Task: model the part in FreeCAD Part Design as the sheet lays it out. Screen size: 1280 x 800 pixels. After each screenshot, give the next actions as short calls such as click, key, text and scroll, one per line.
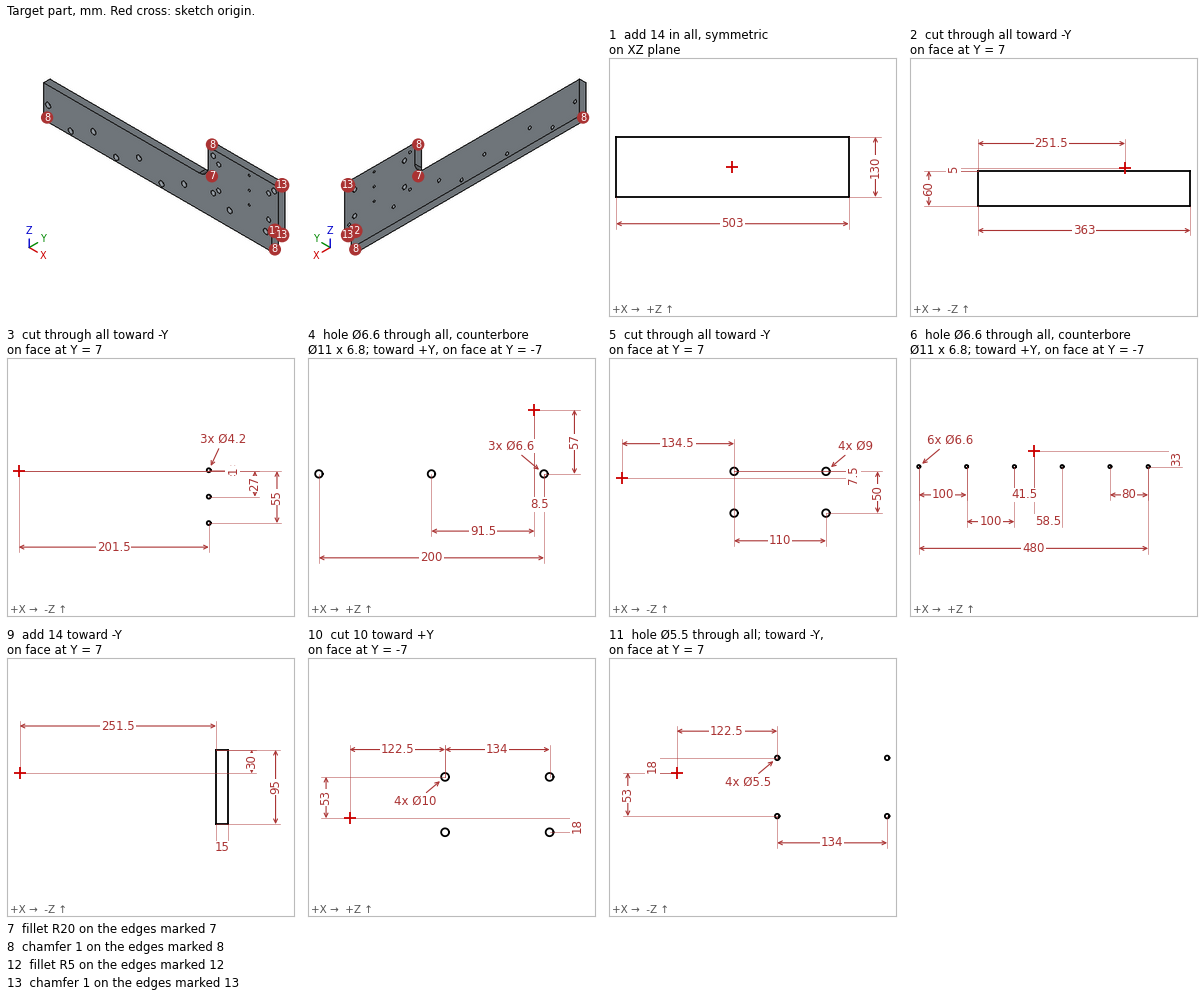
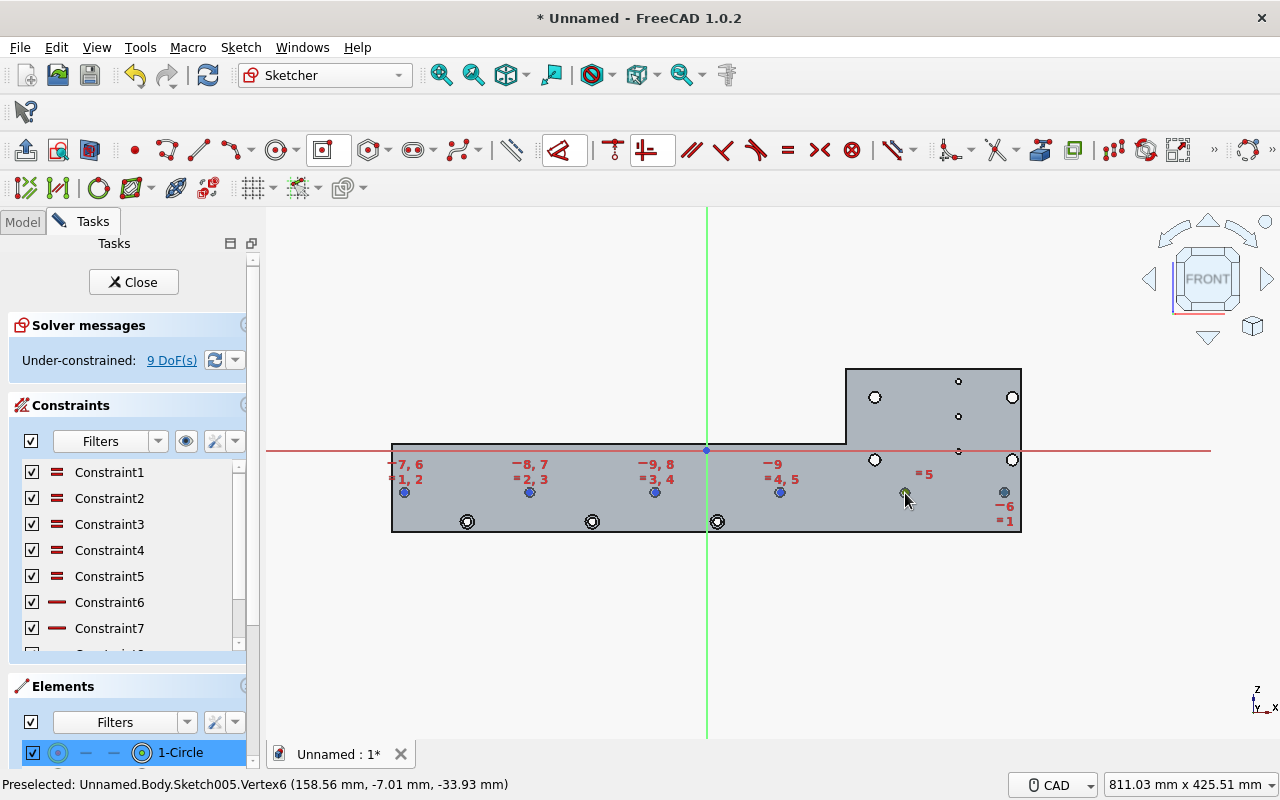
key(h)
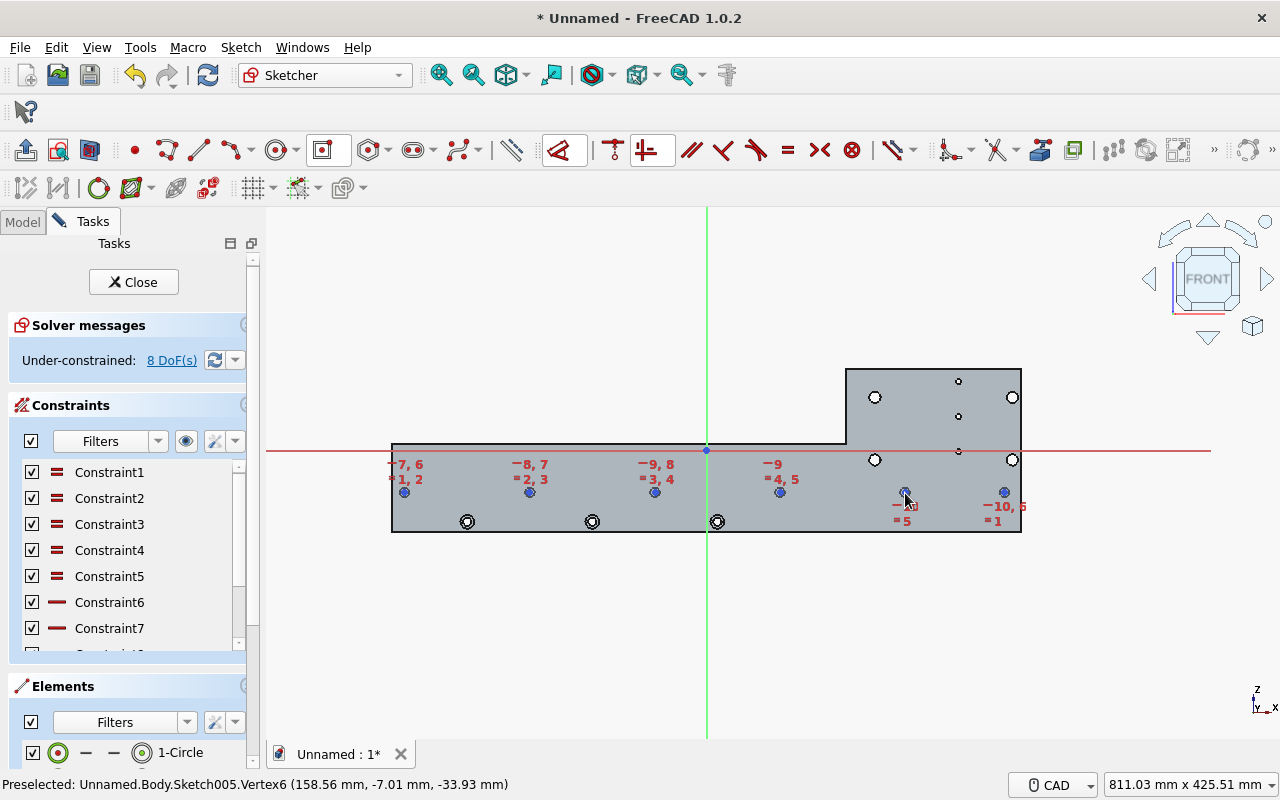
scroll(1000, 492, up, 8)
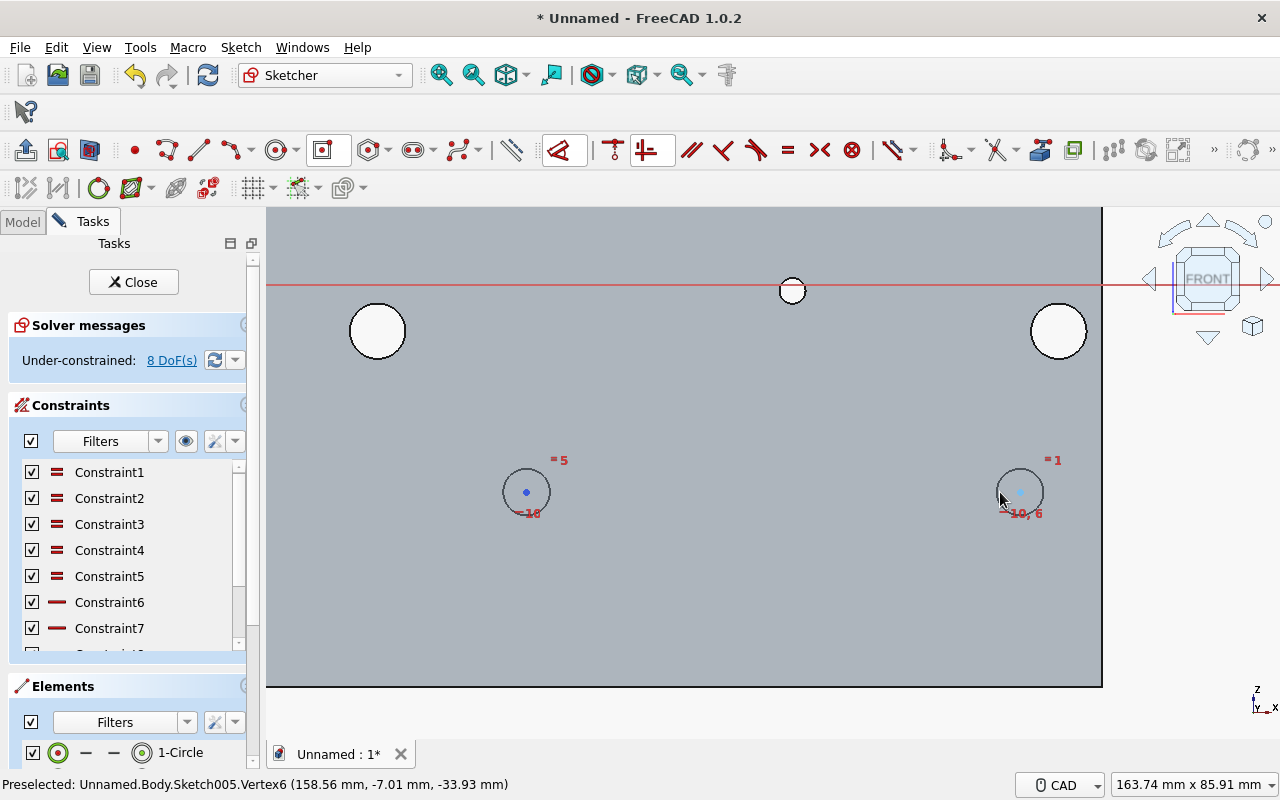
click(997, 491)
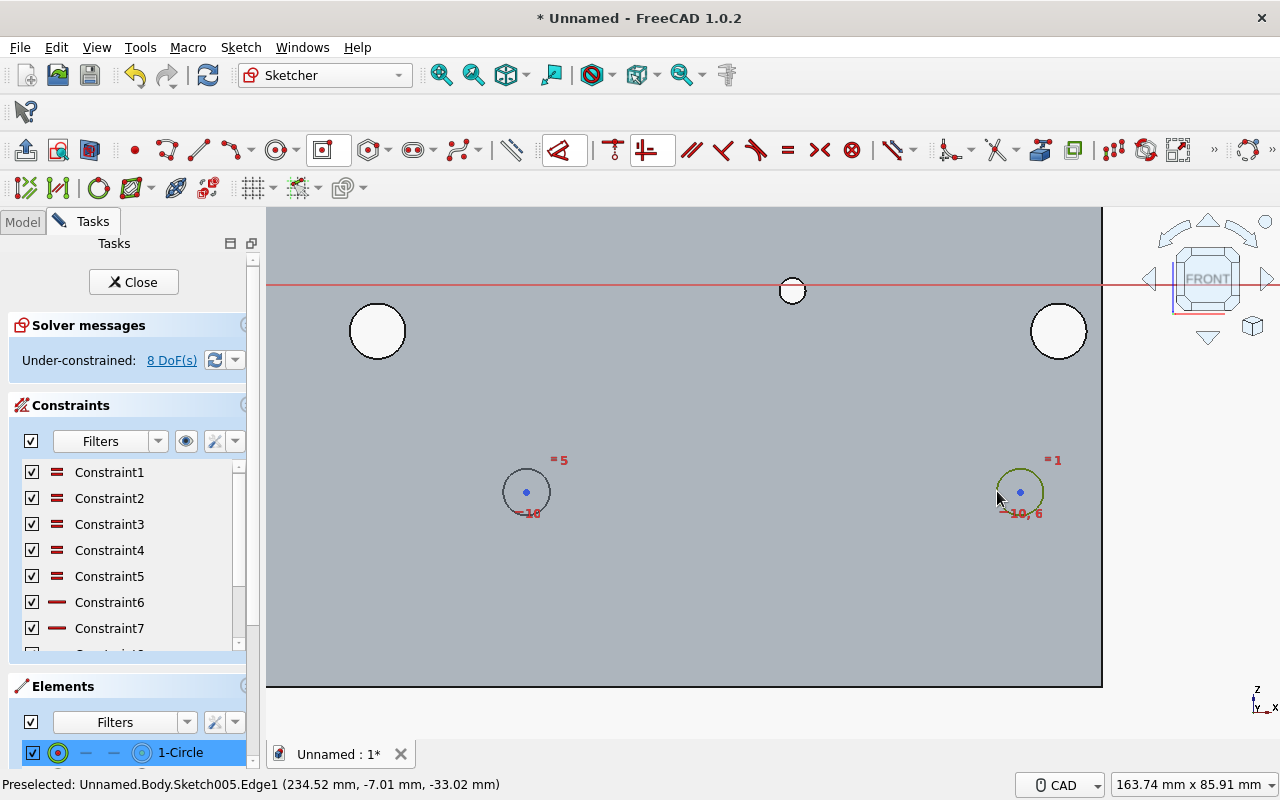
key(k)
key(o)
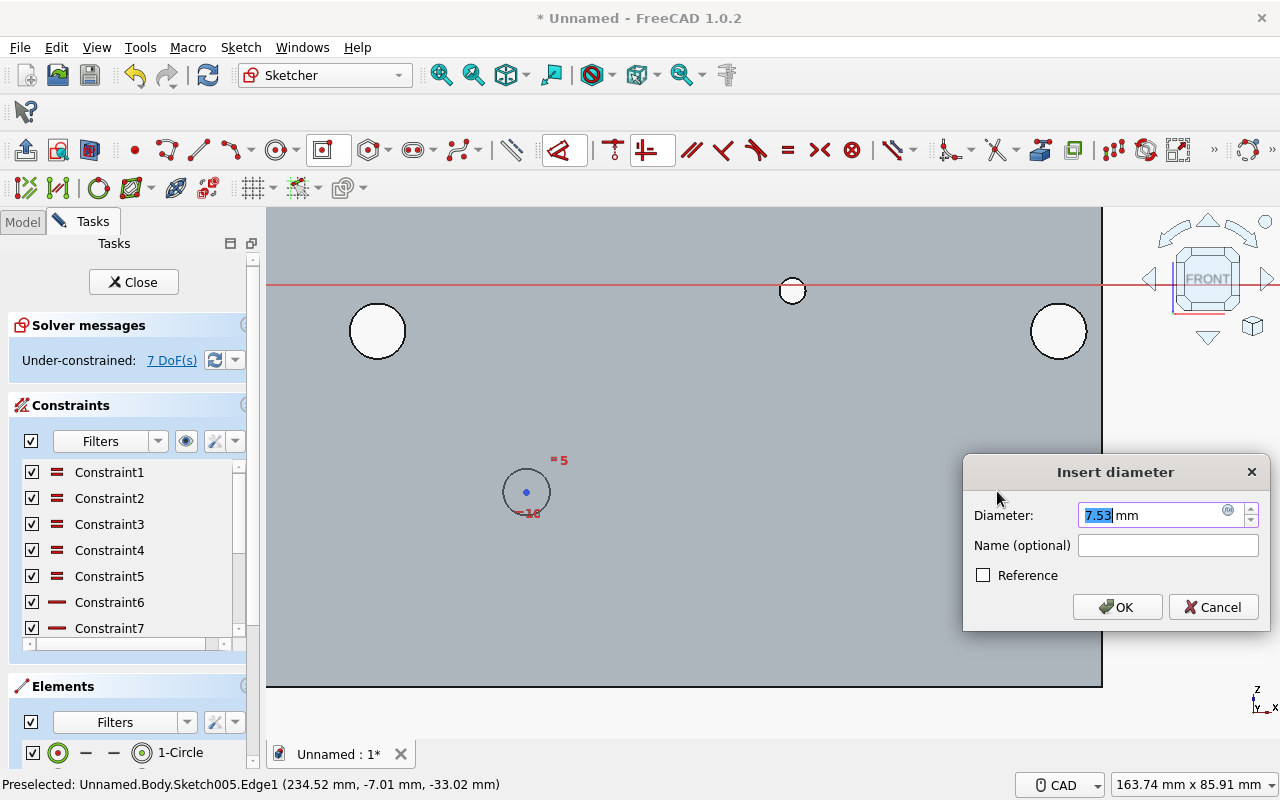
text(6.6)
key(Return)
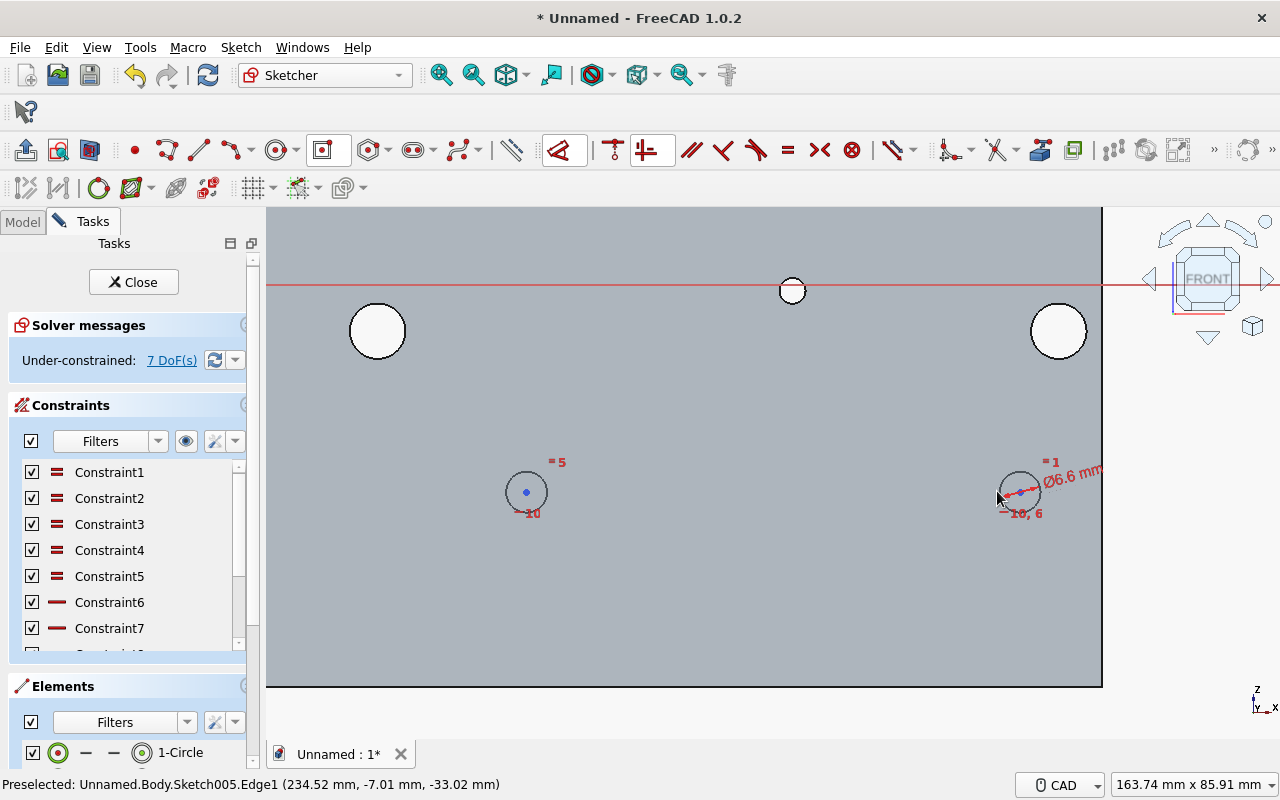
scroll(1000, 492, down, 8)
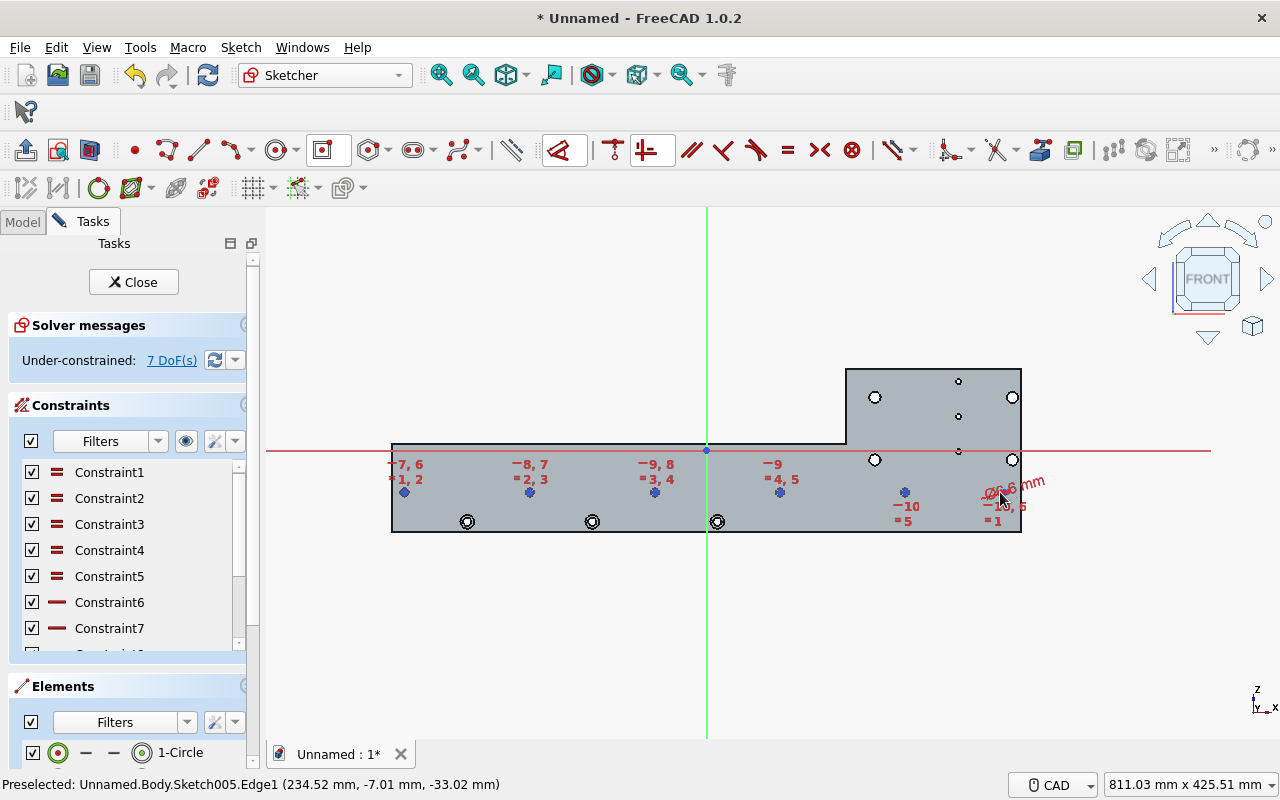
click(1005, 492)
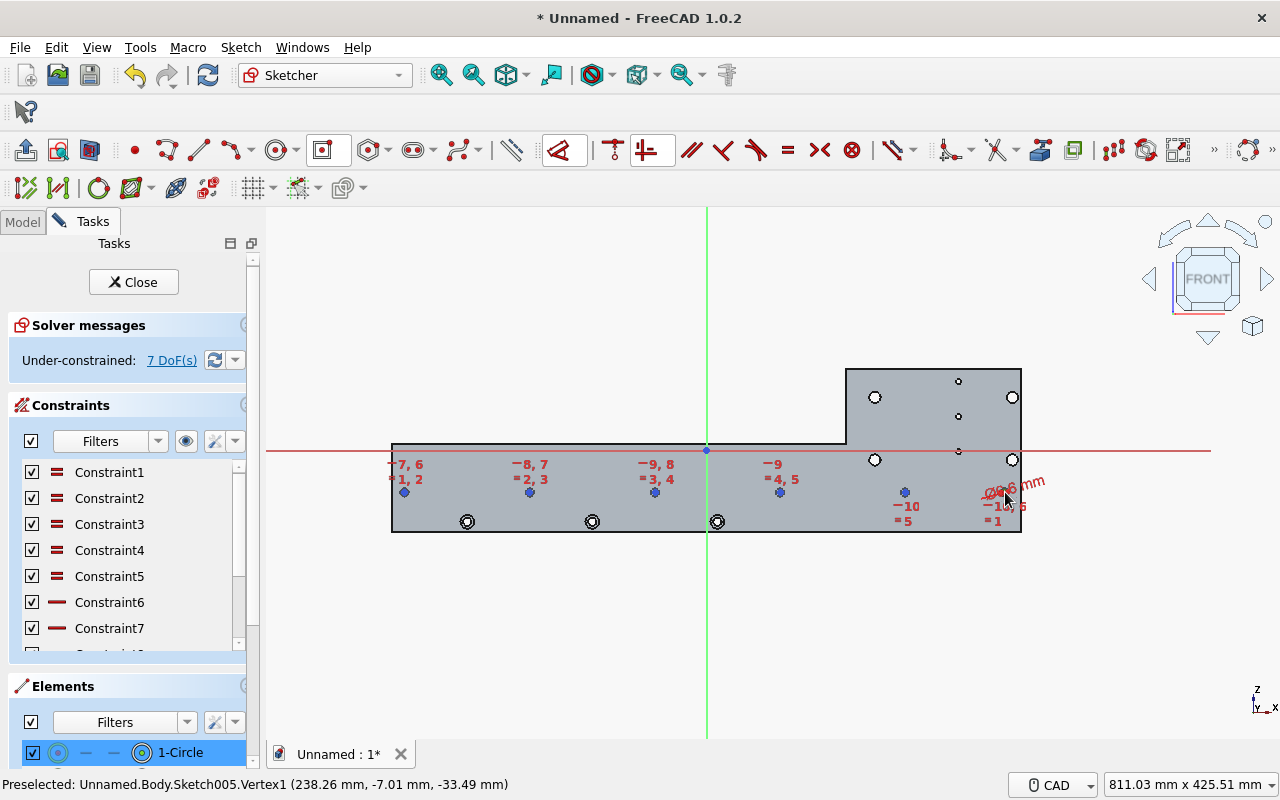
key(i)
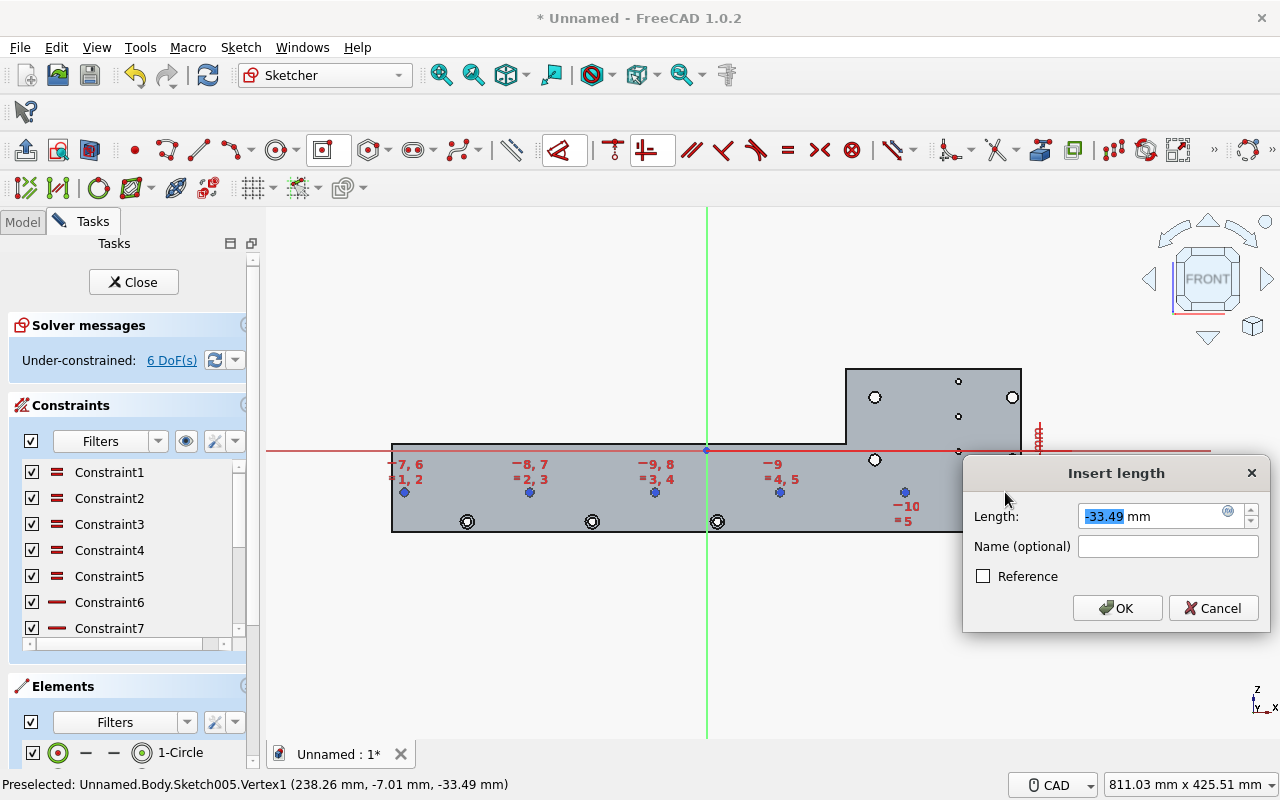
text(-33)
key(Return)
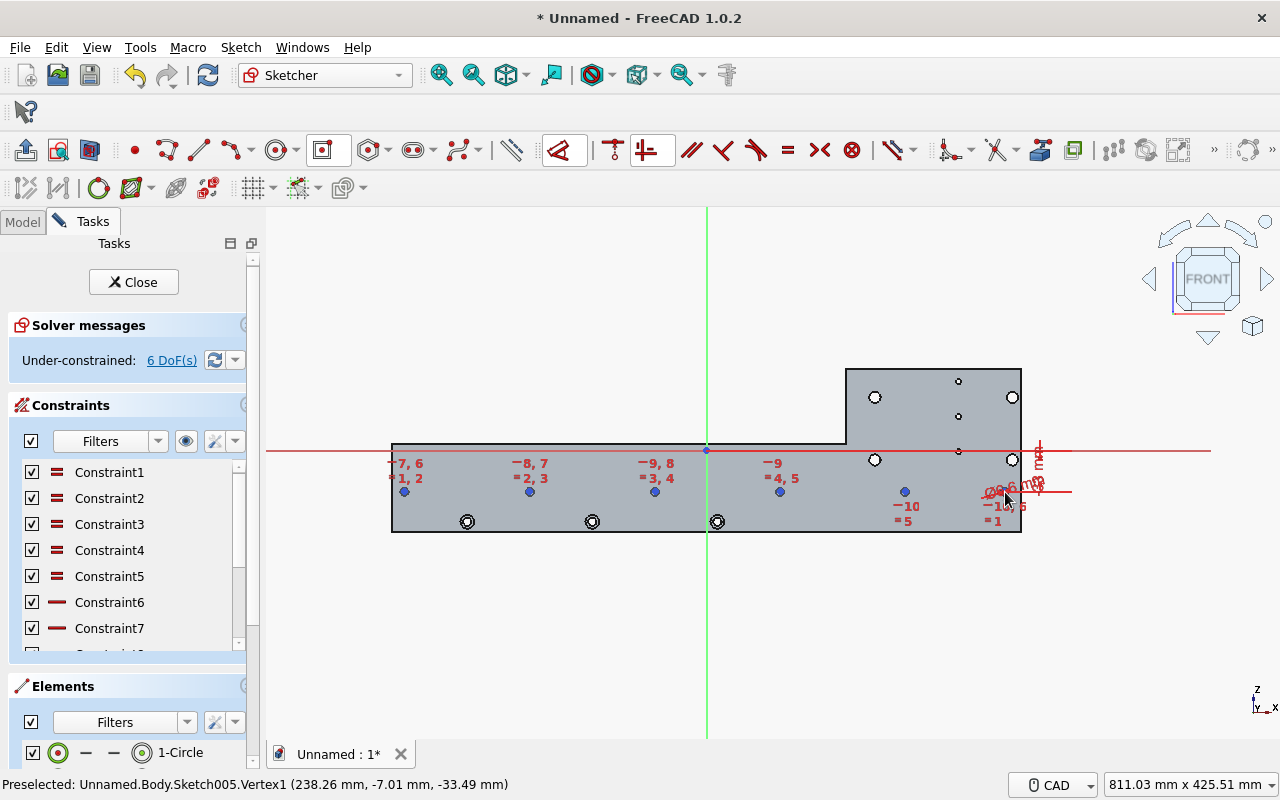
click(1005, 492)